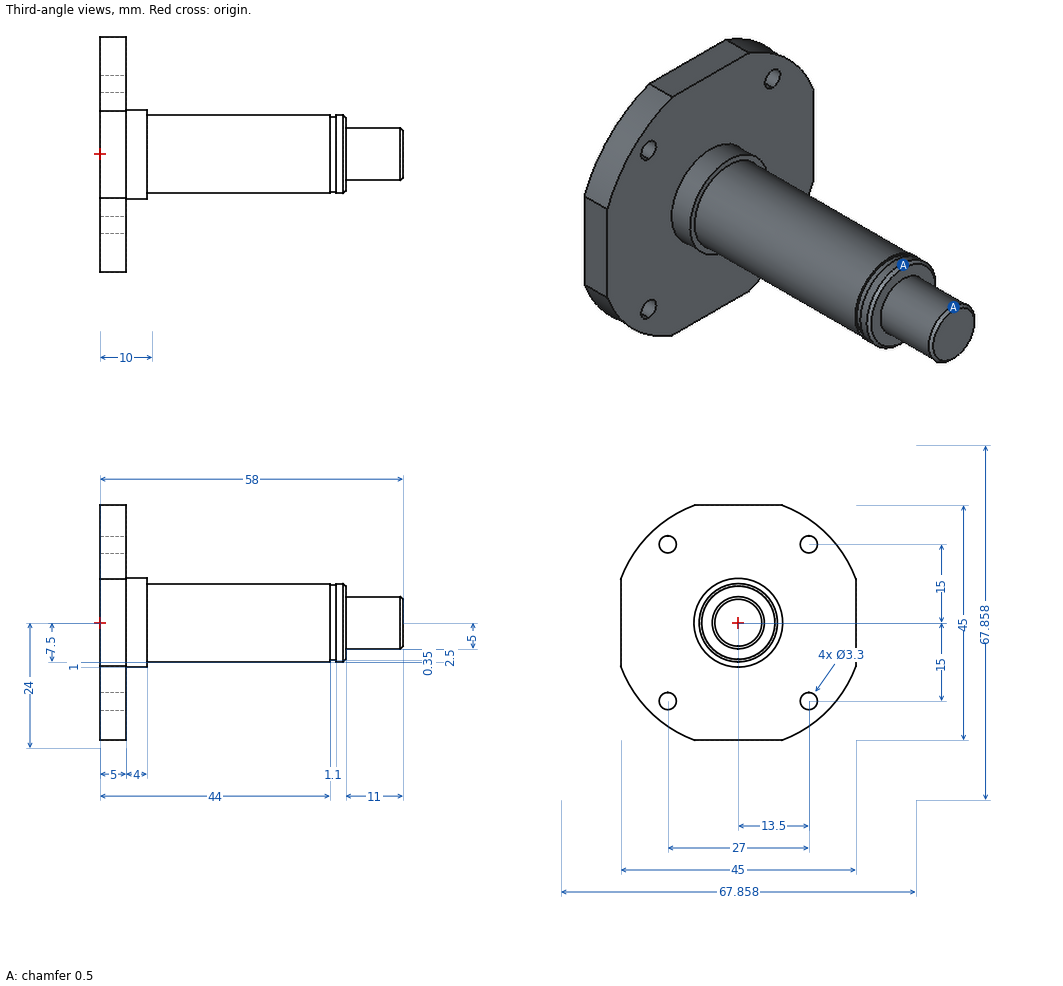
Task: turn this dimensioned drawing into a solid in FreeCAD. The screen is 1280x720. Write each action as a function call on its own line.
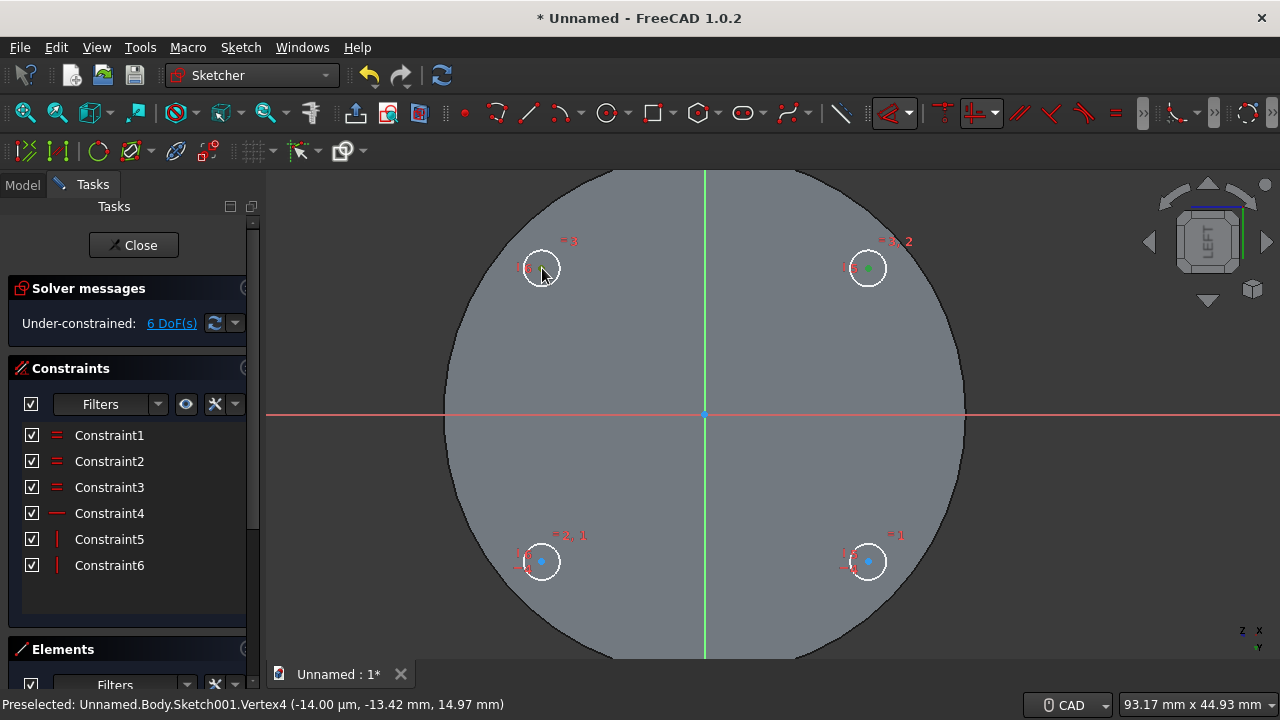
click(998, 114)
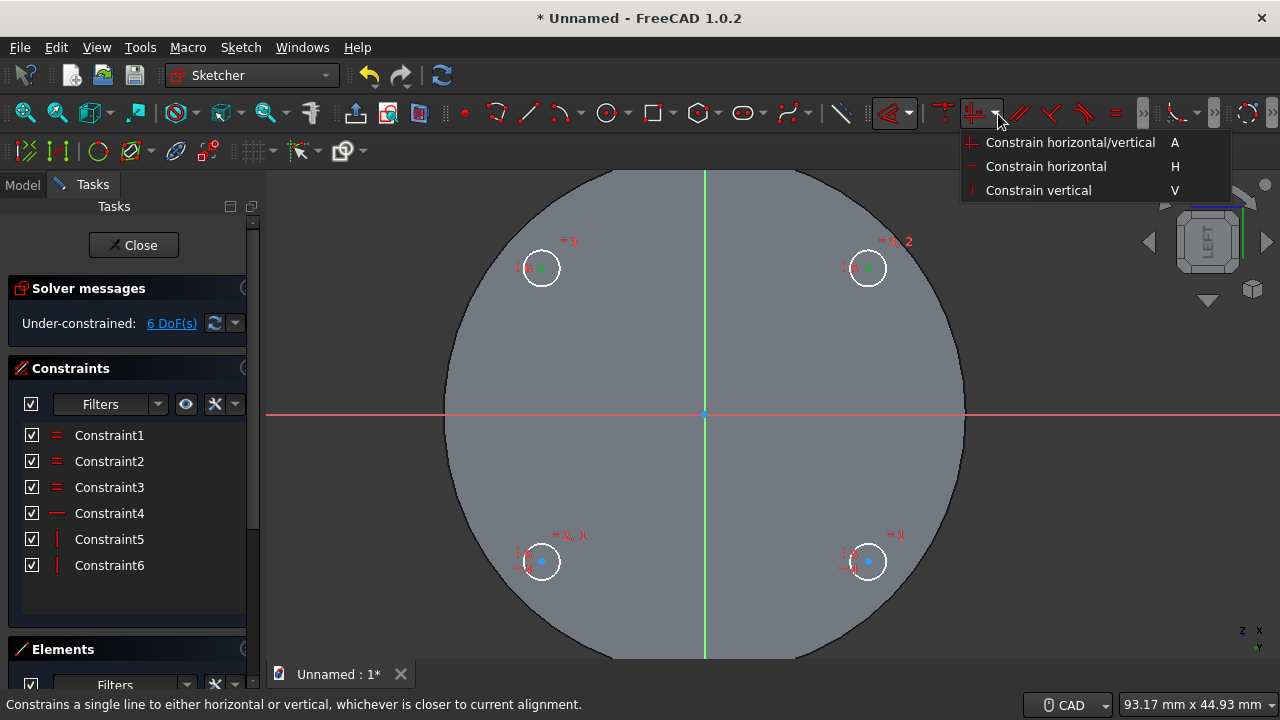
click(1096, 166)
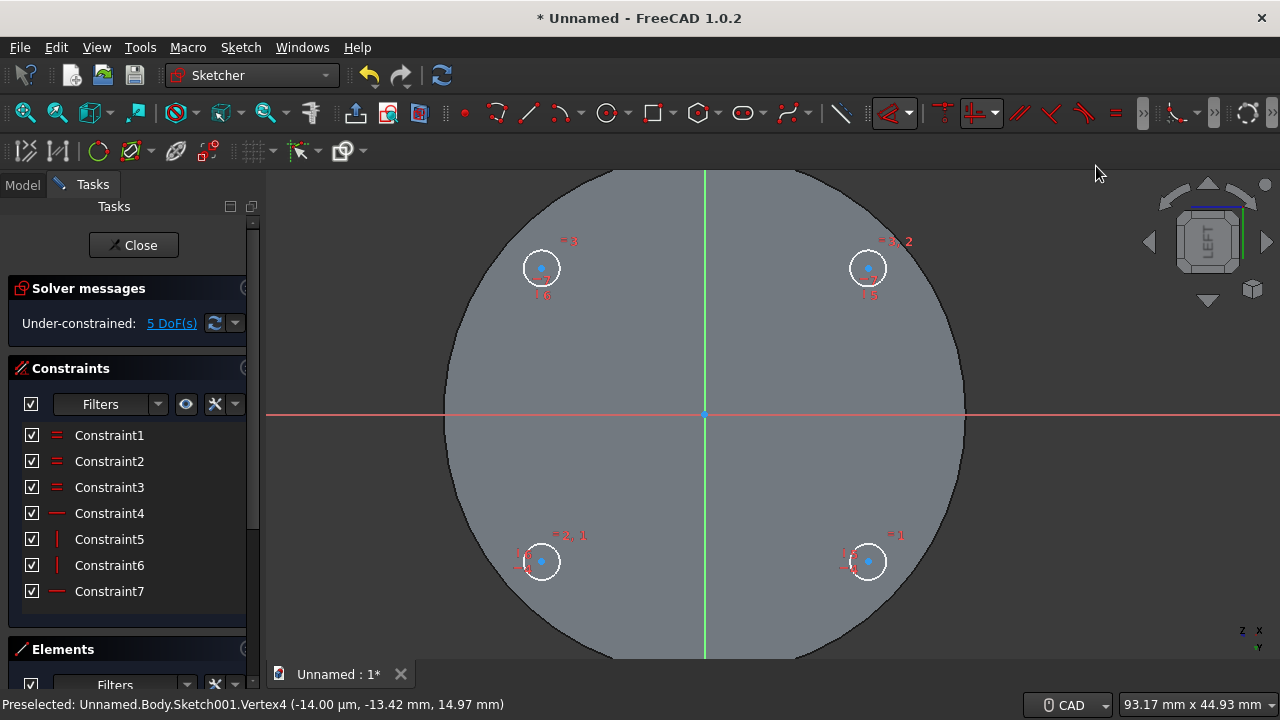
click(881, 549)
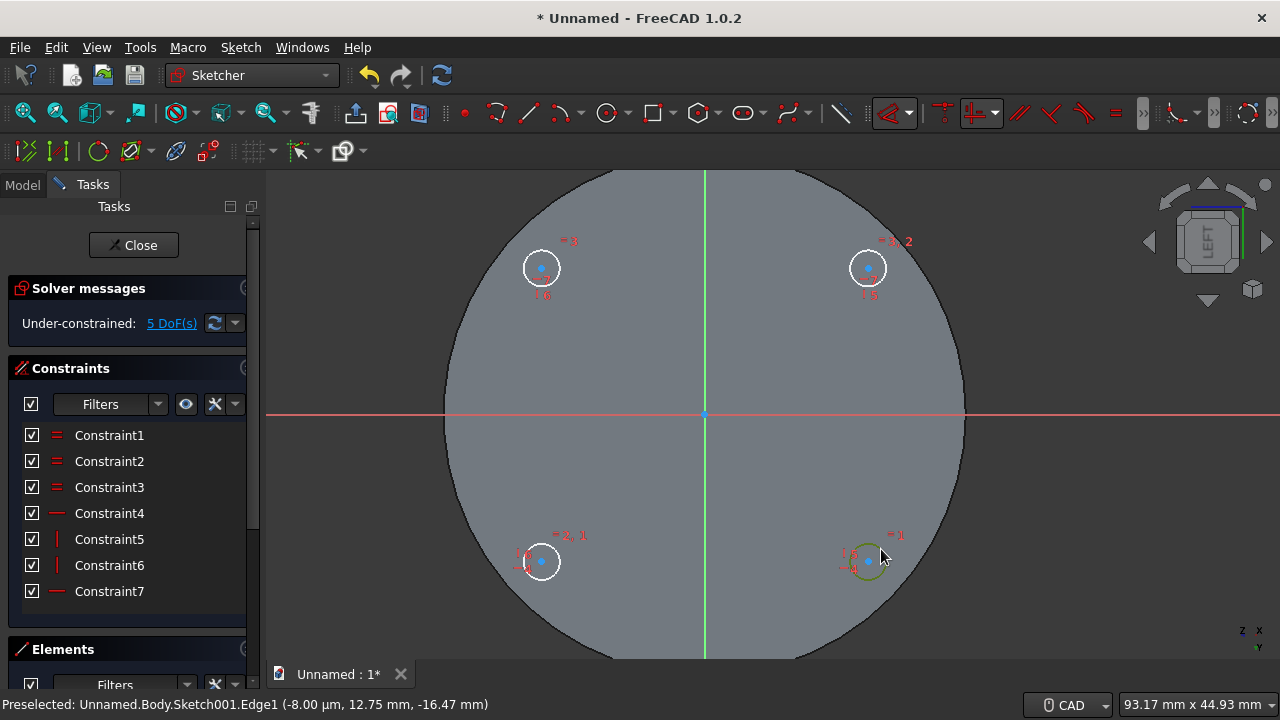
click(912, 114)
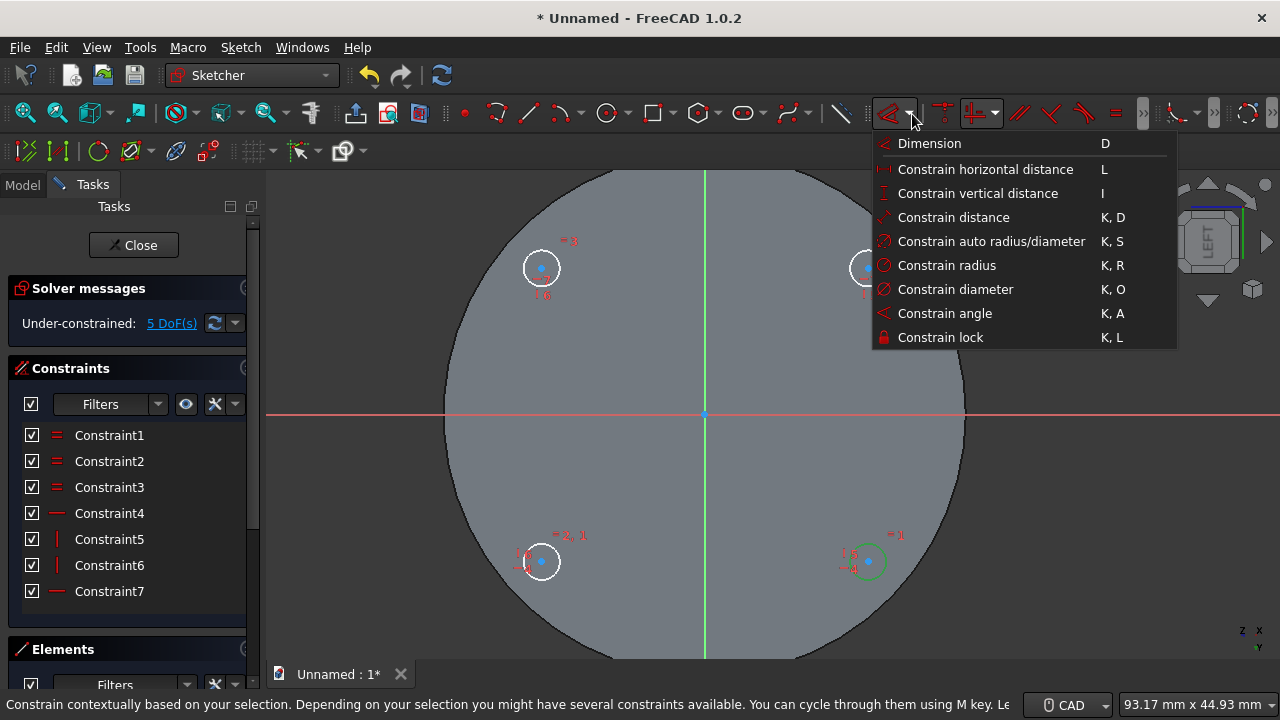
click(1025, 289)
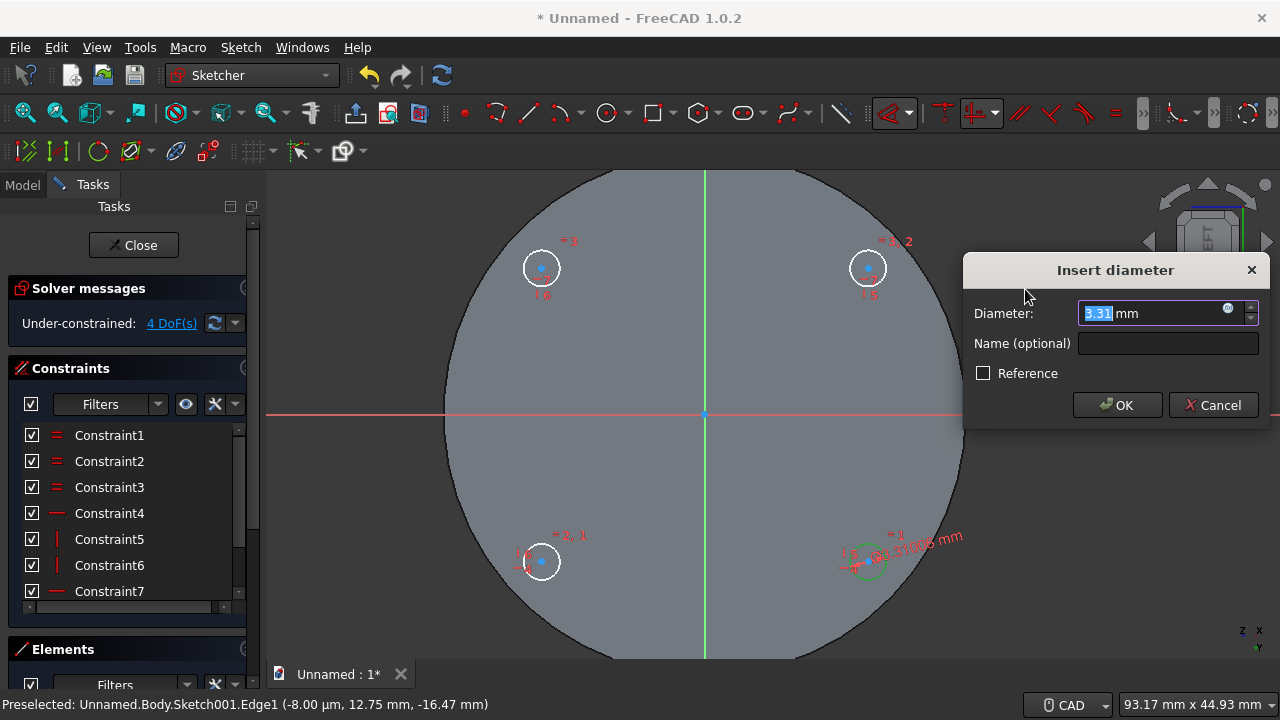
text(3.3)
key(Return)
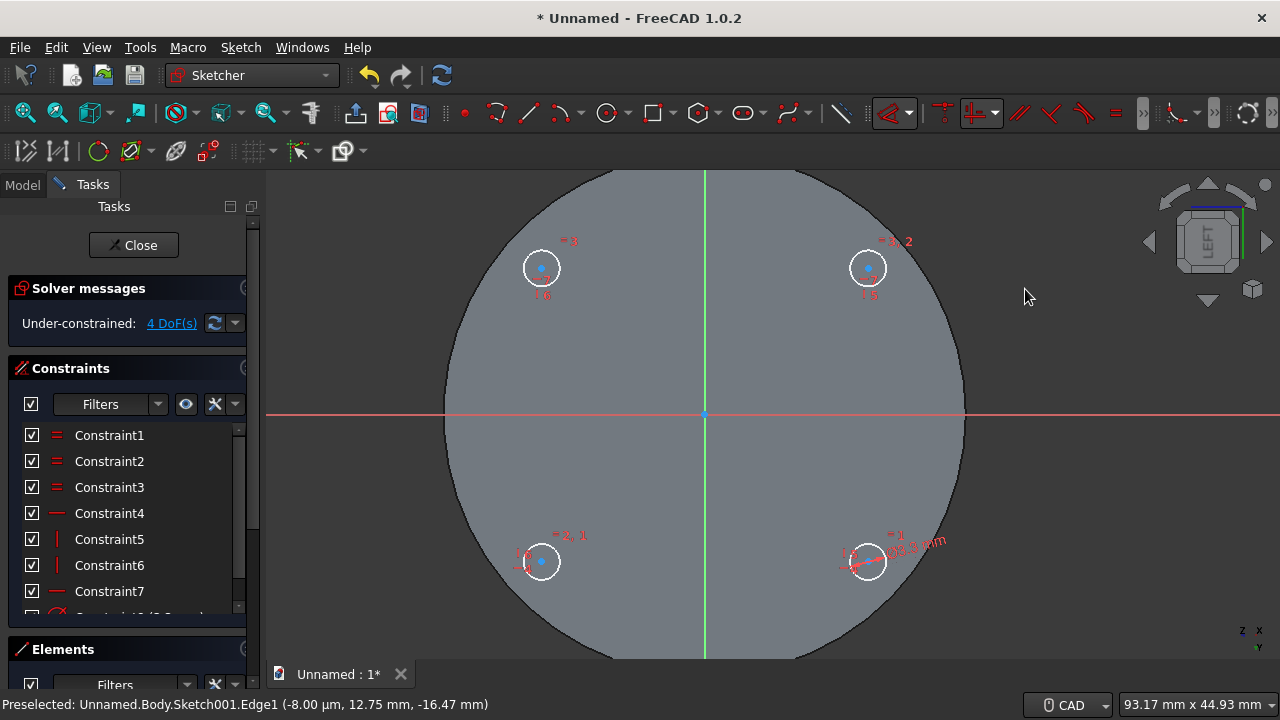
click(868, 562)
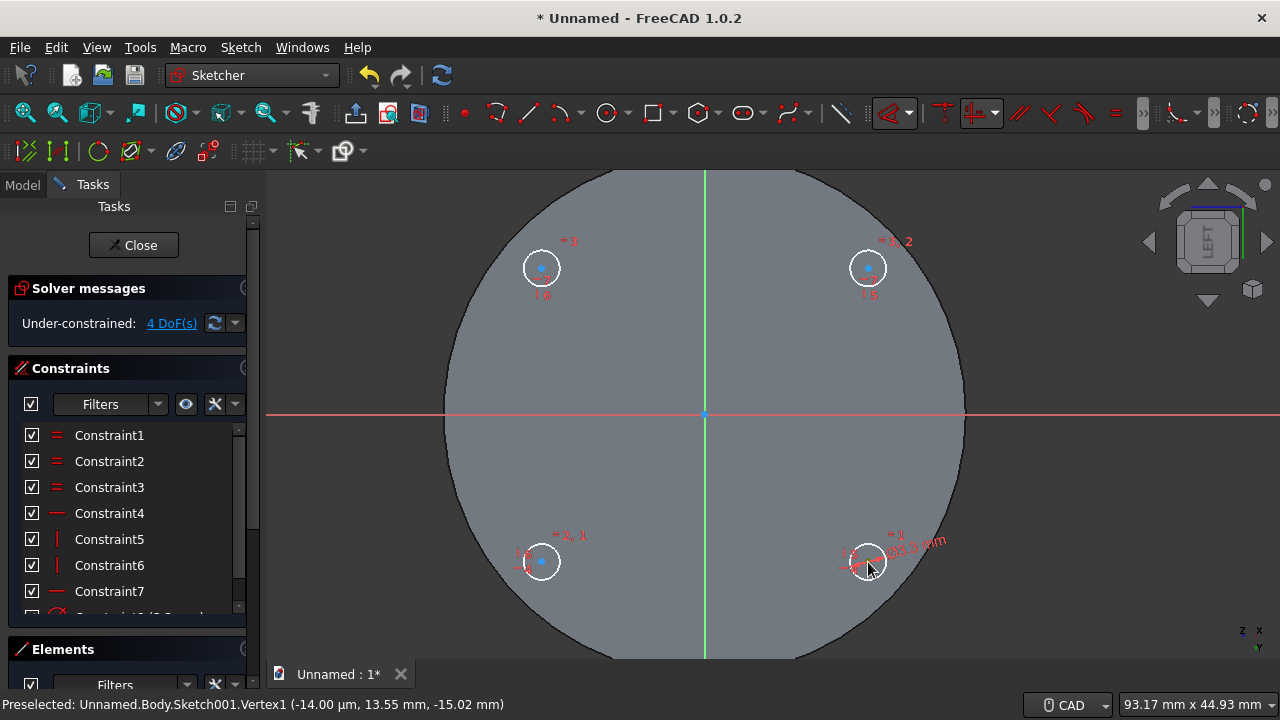
click(912, 114)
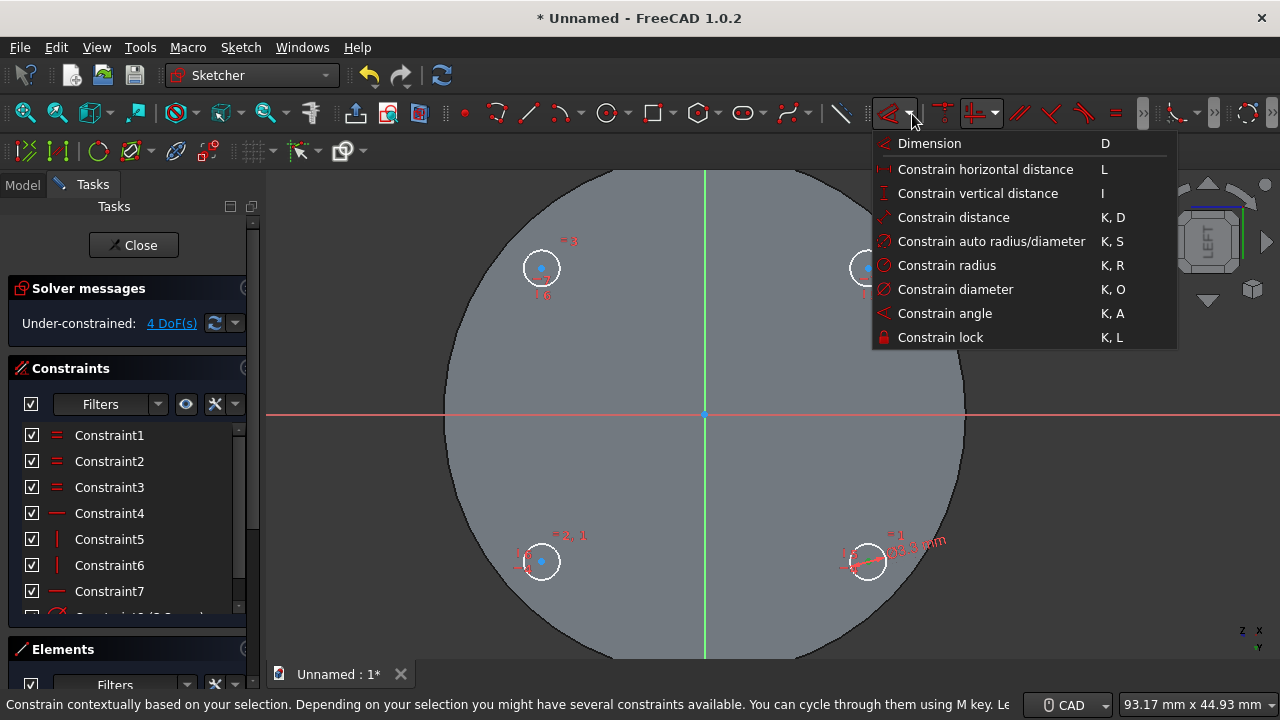
click(1025, 169)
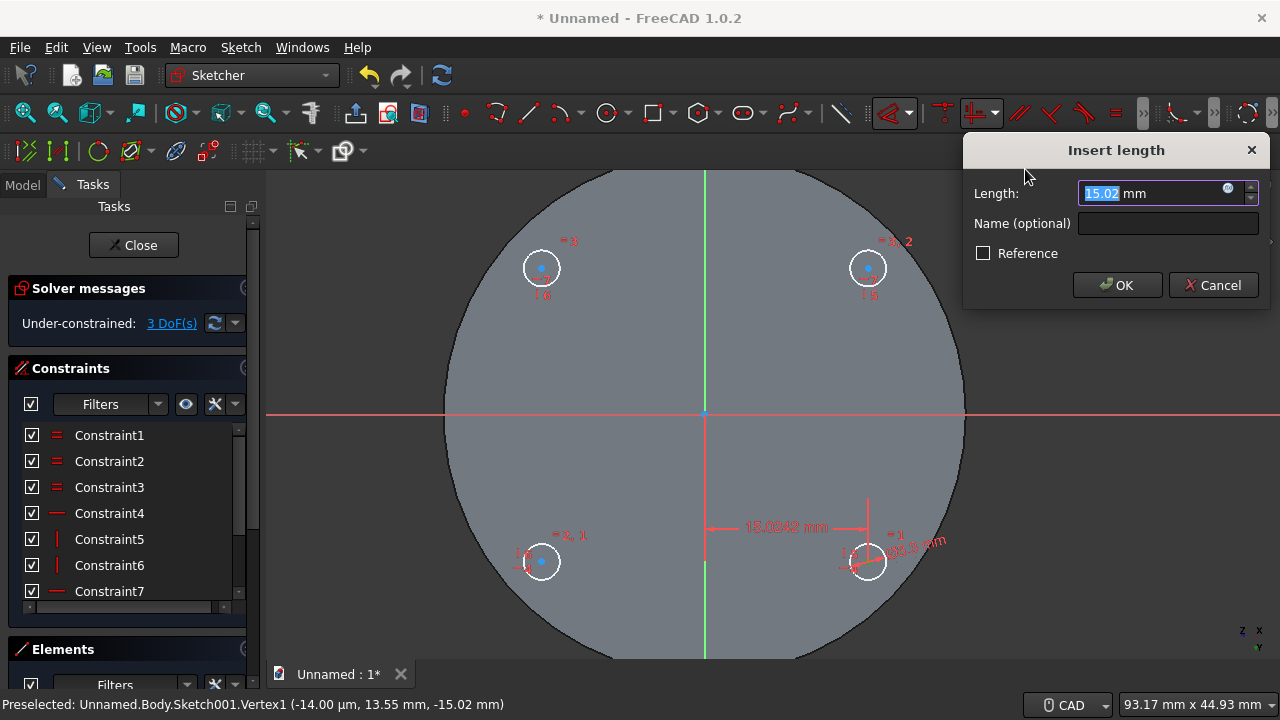
text(15)
key(Return)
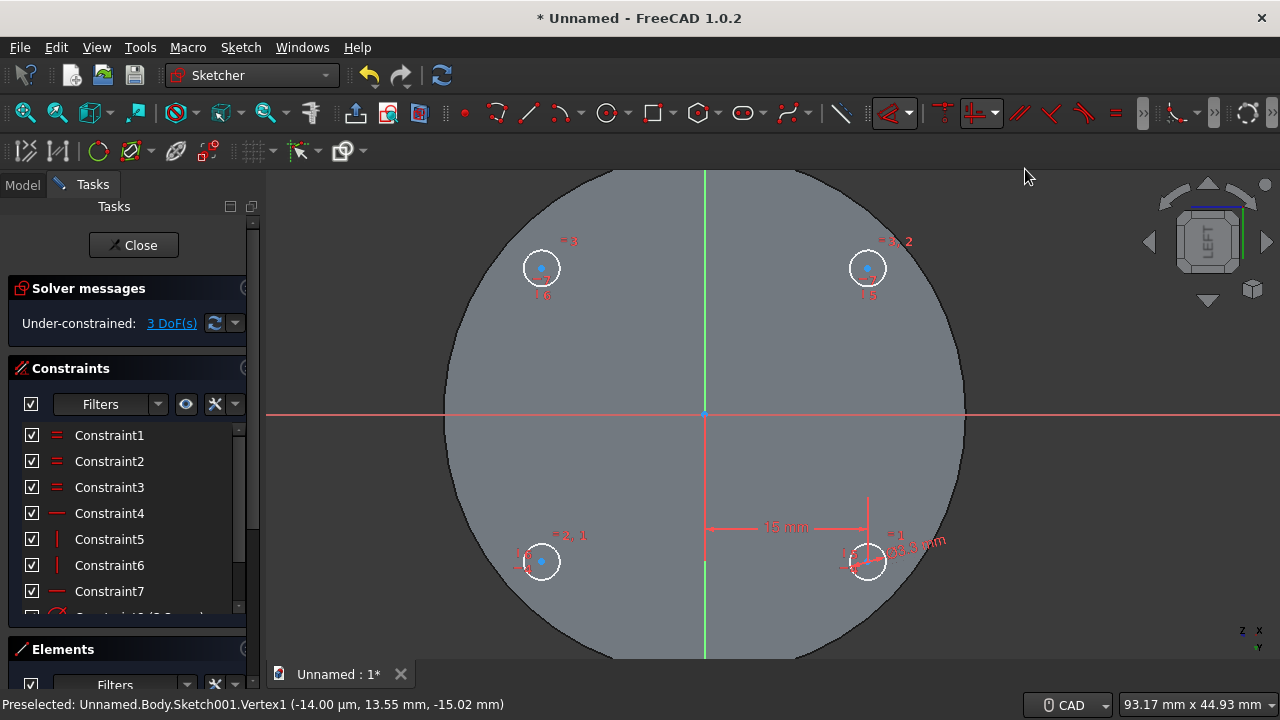
click(542, 562)